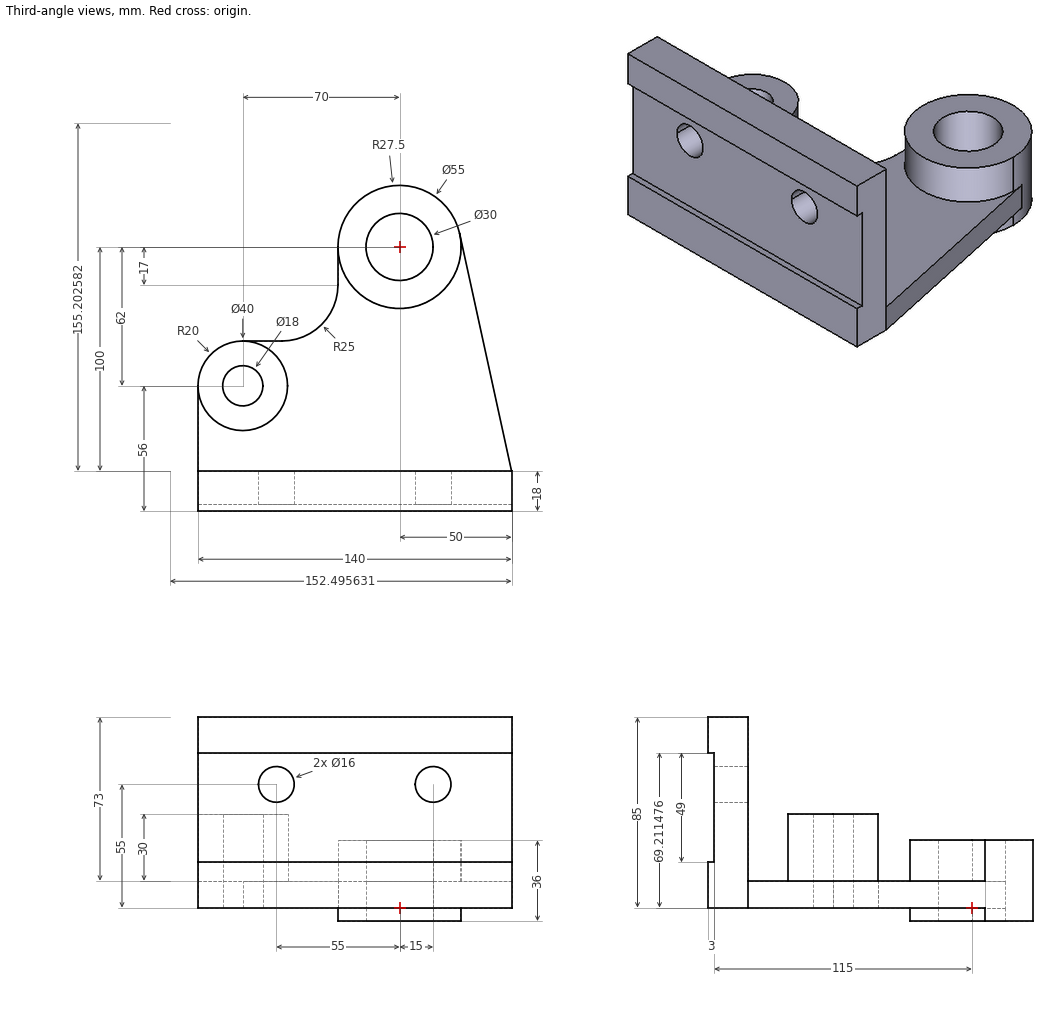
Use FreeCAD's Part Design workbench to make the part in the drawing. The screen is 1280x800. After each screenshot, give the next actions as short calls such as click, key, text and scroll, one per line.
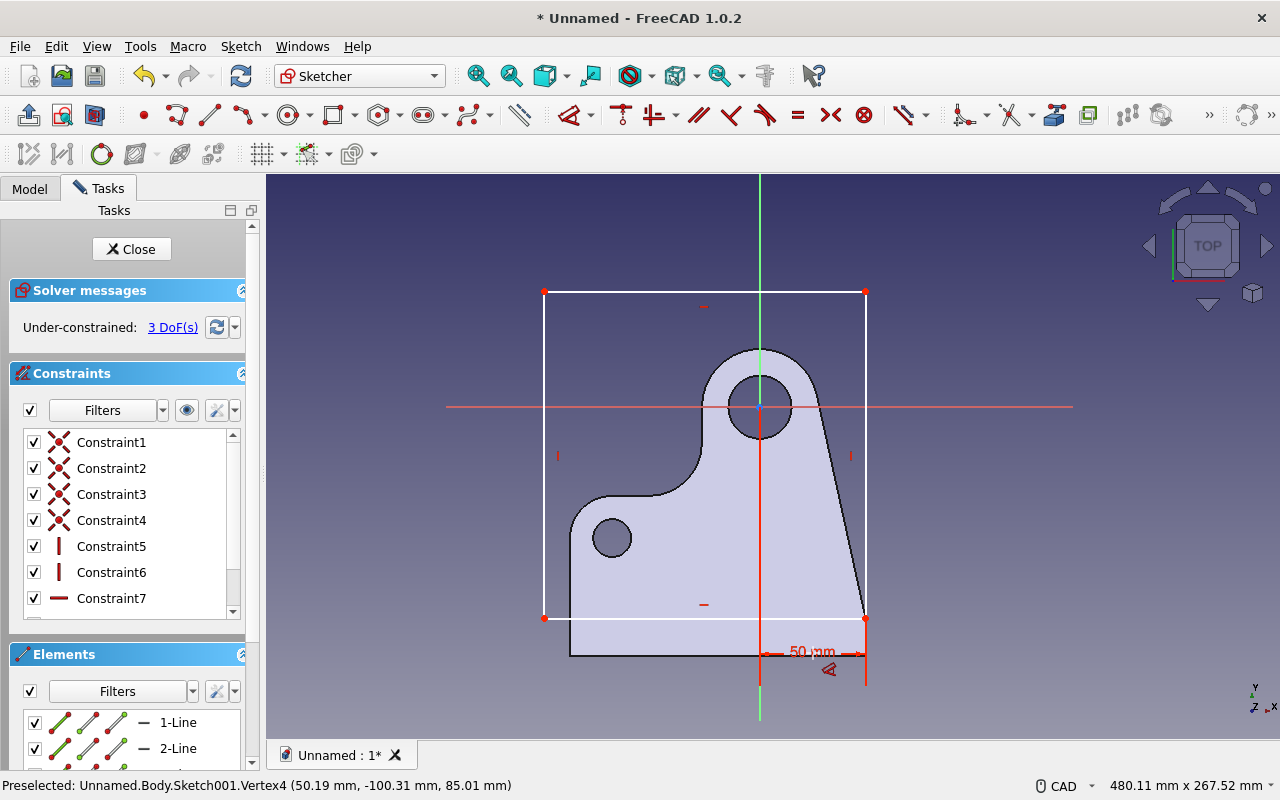
click(544, 619)
click(510, 513)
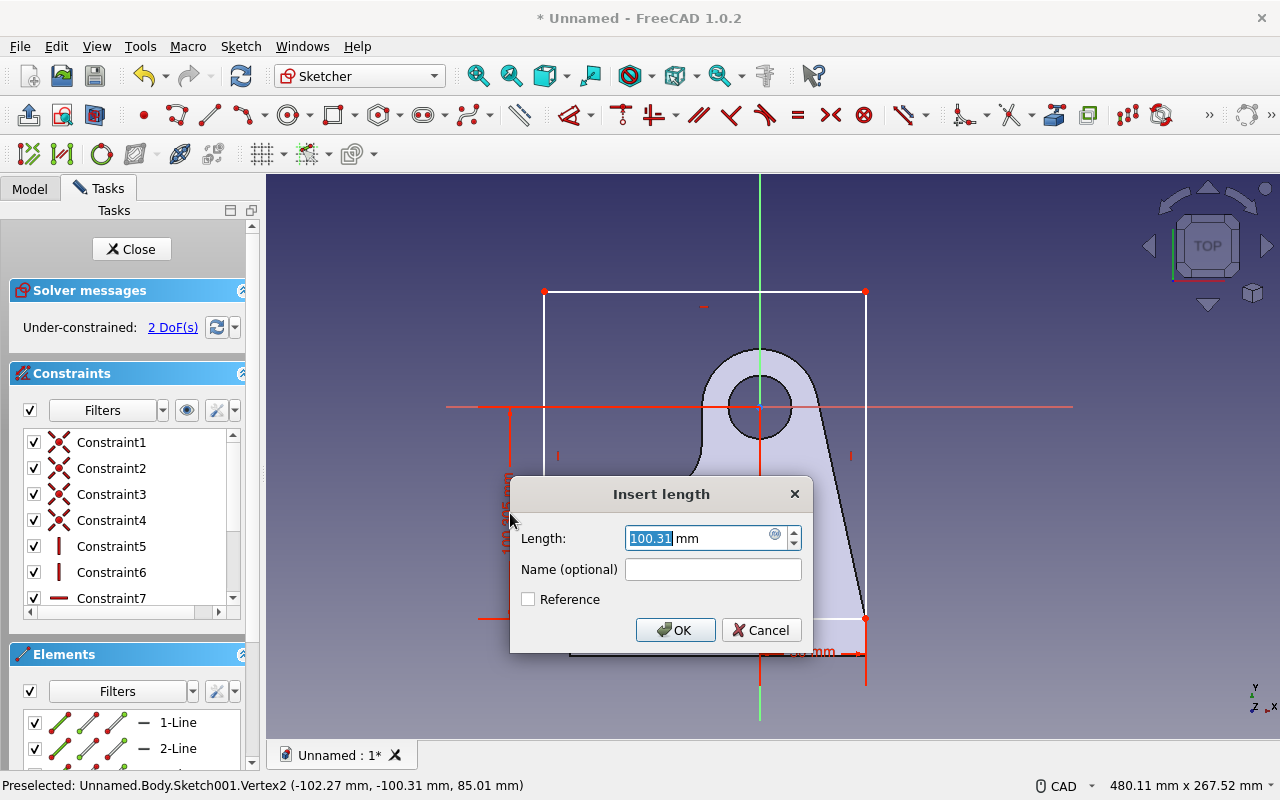
text(100)
key(Return)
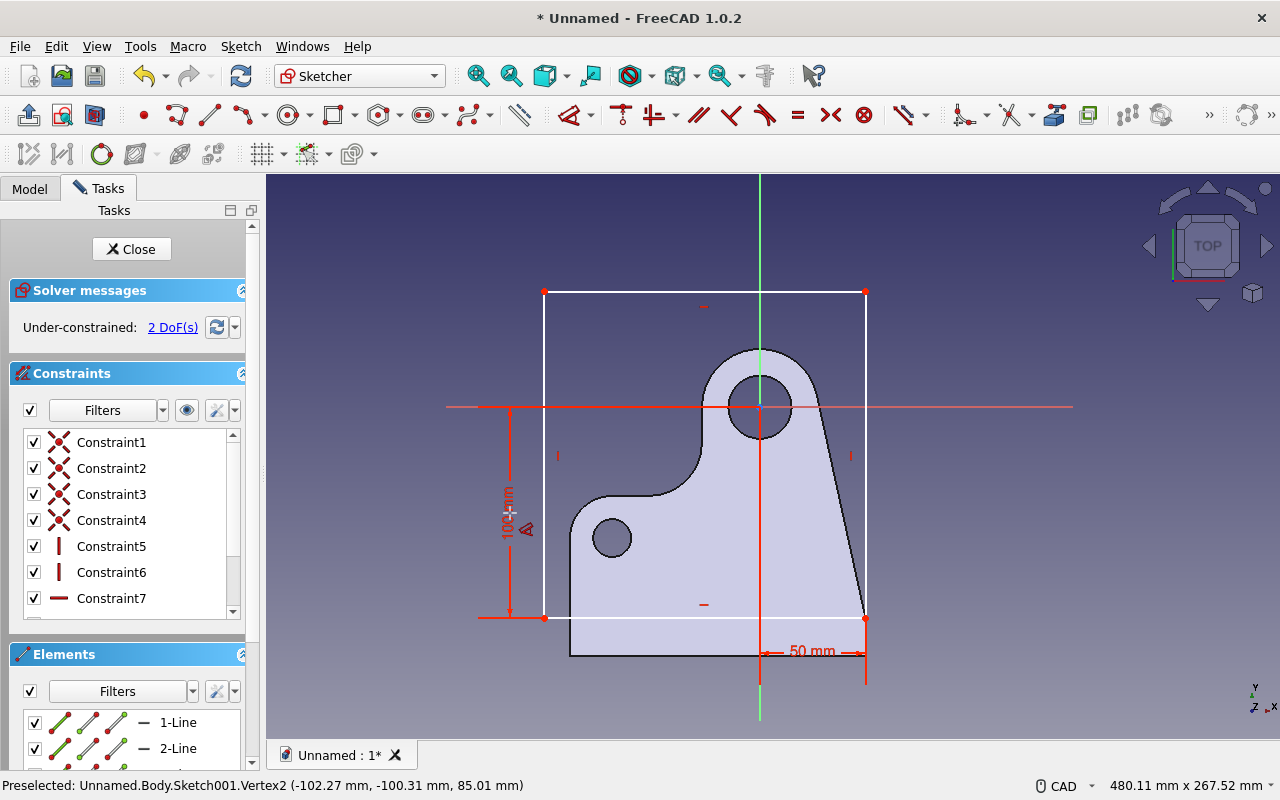
click(544, 390)
click(510, 455)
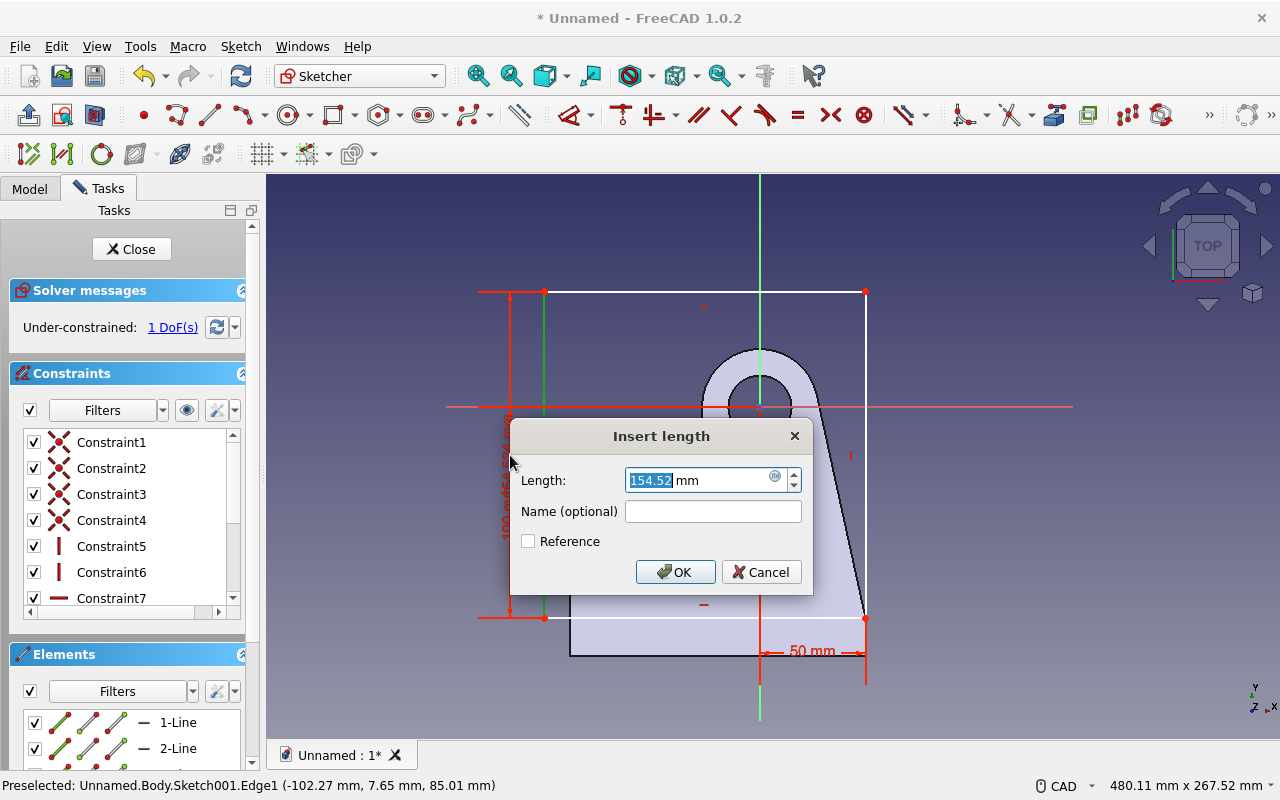
text(155.202582)
key(Return)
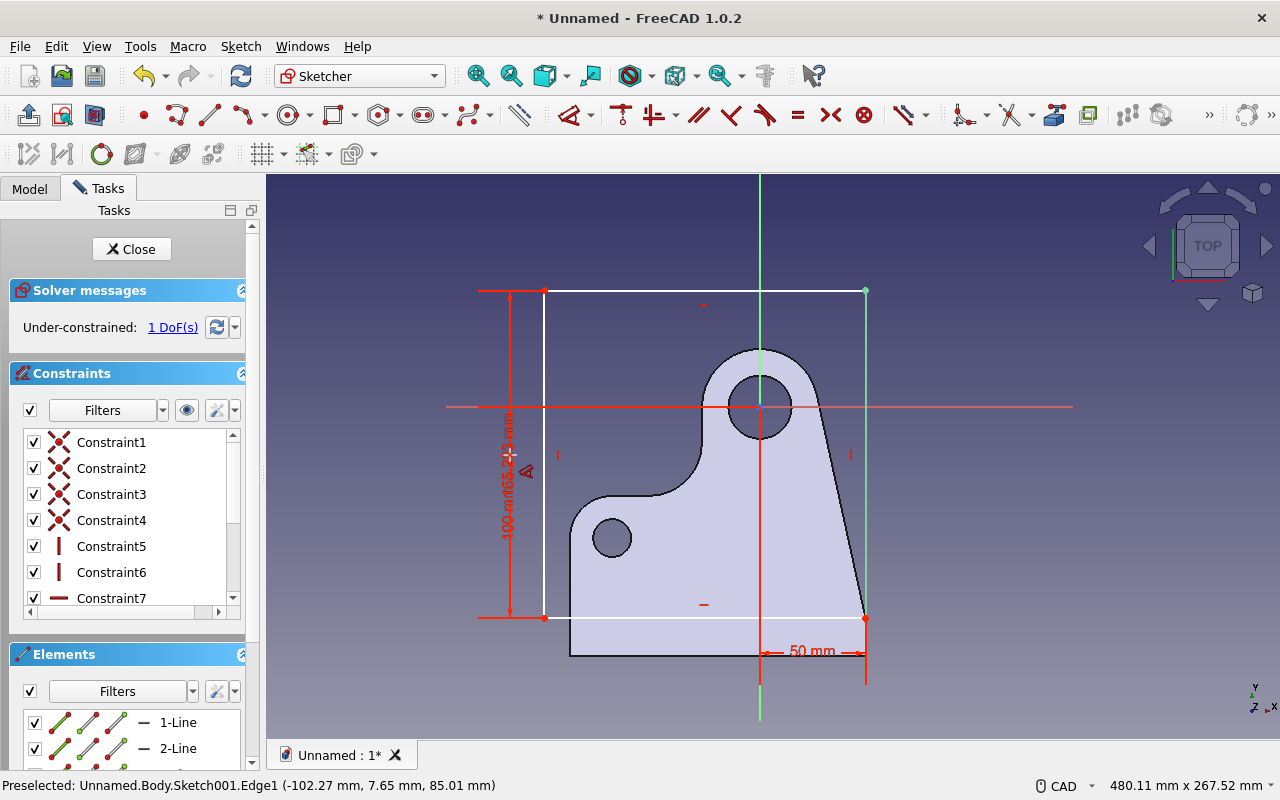
click(640, 618)
click(705, 652)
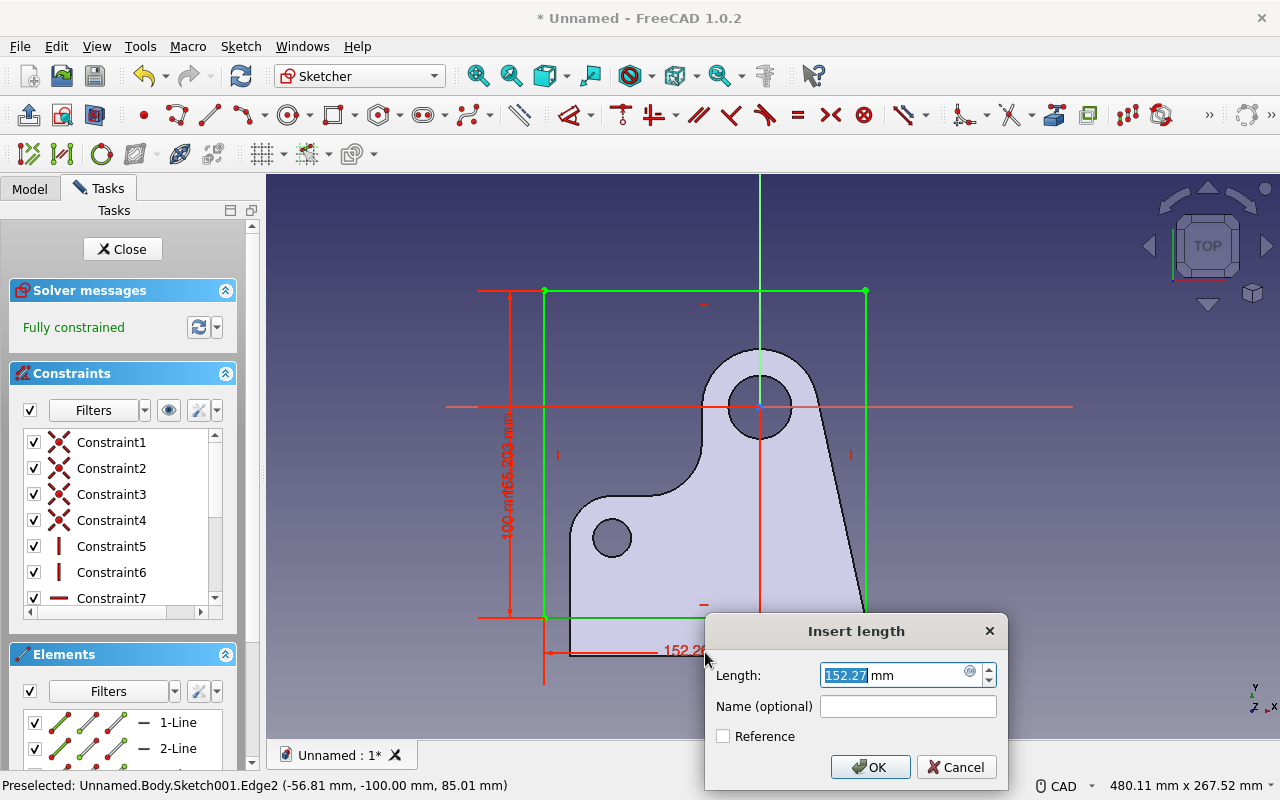
text(152.495631)
key(Return)
key(Escape)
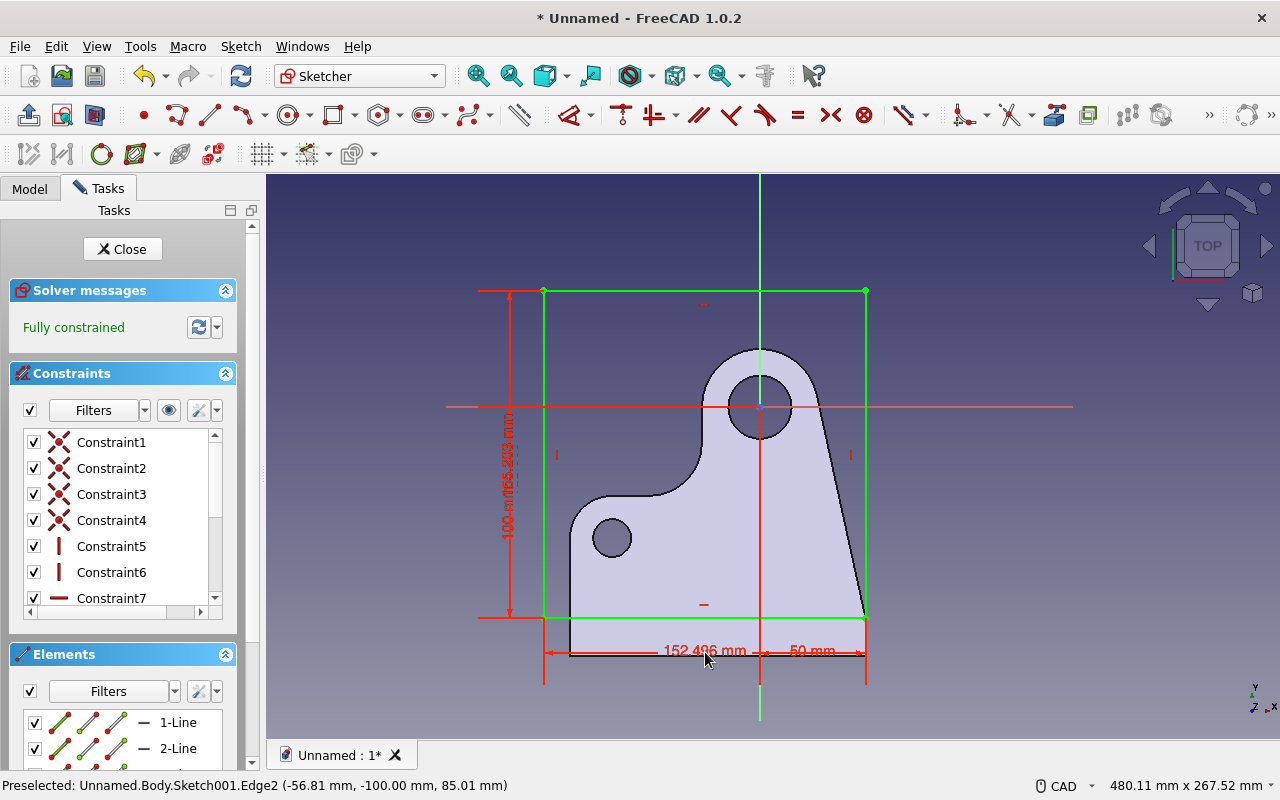
click(123, 249)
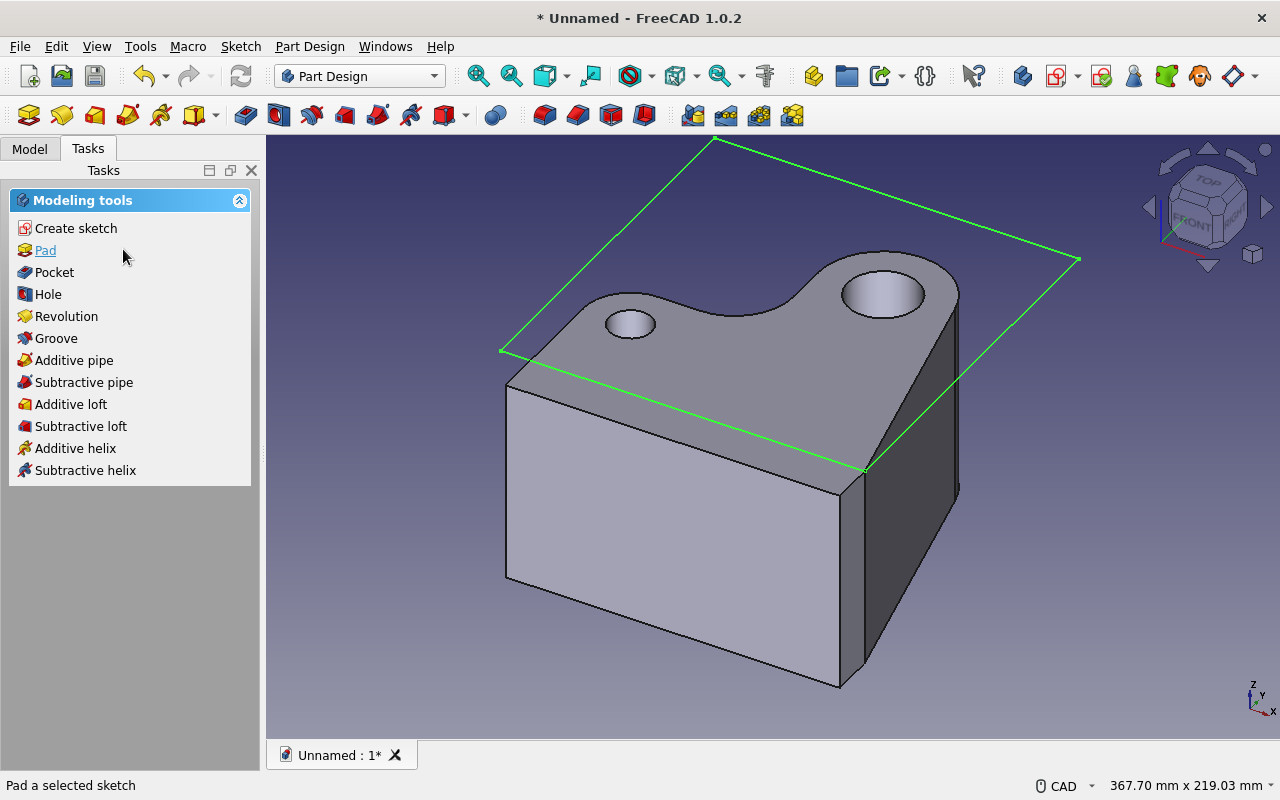
click(246, 116)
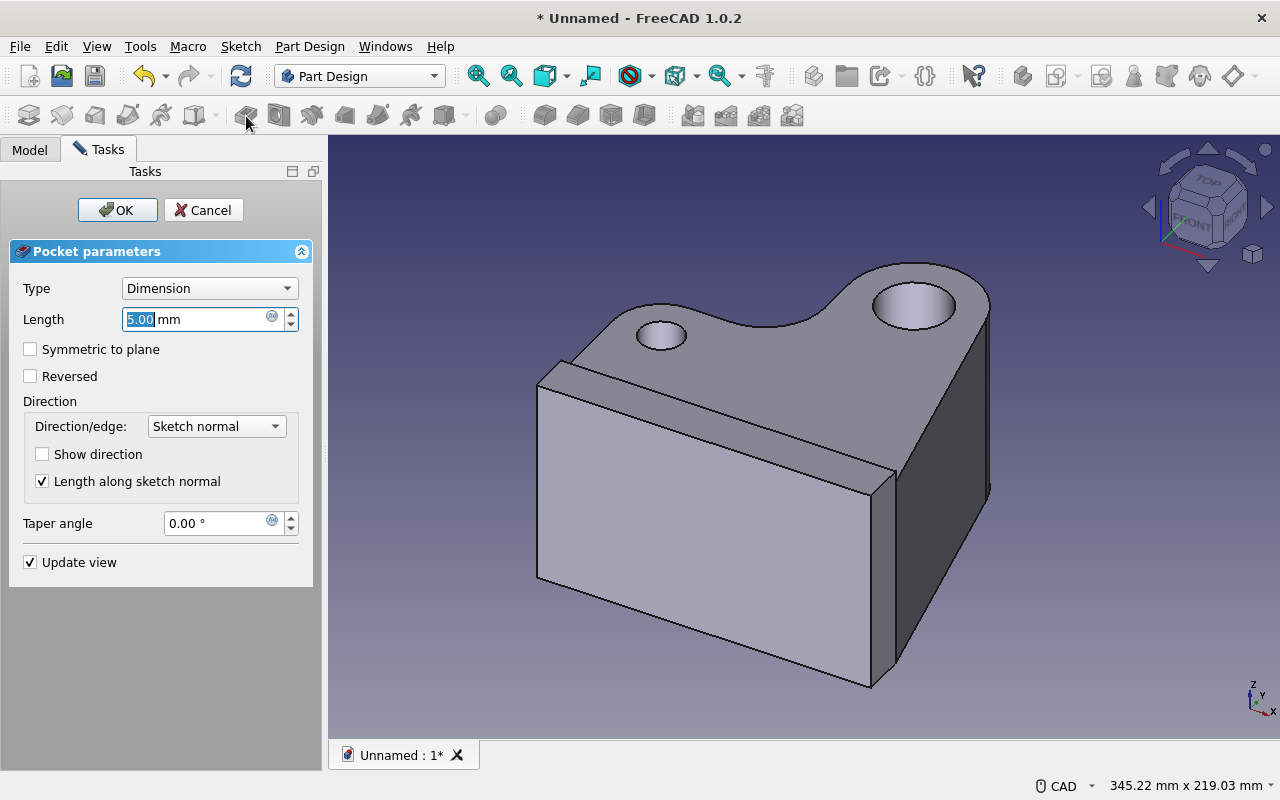
text(73)
key(Tab)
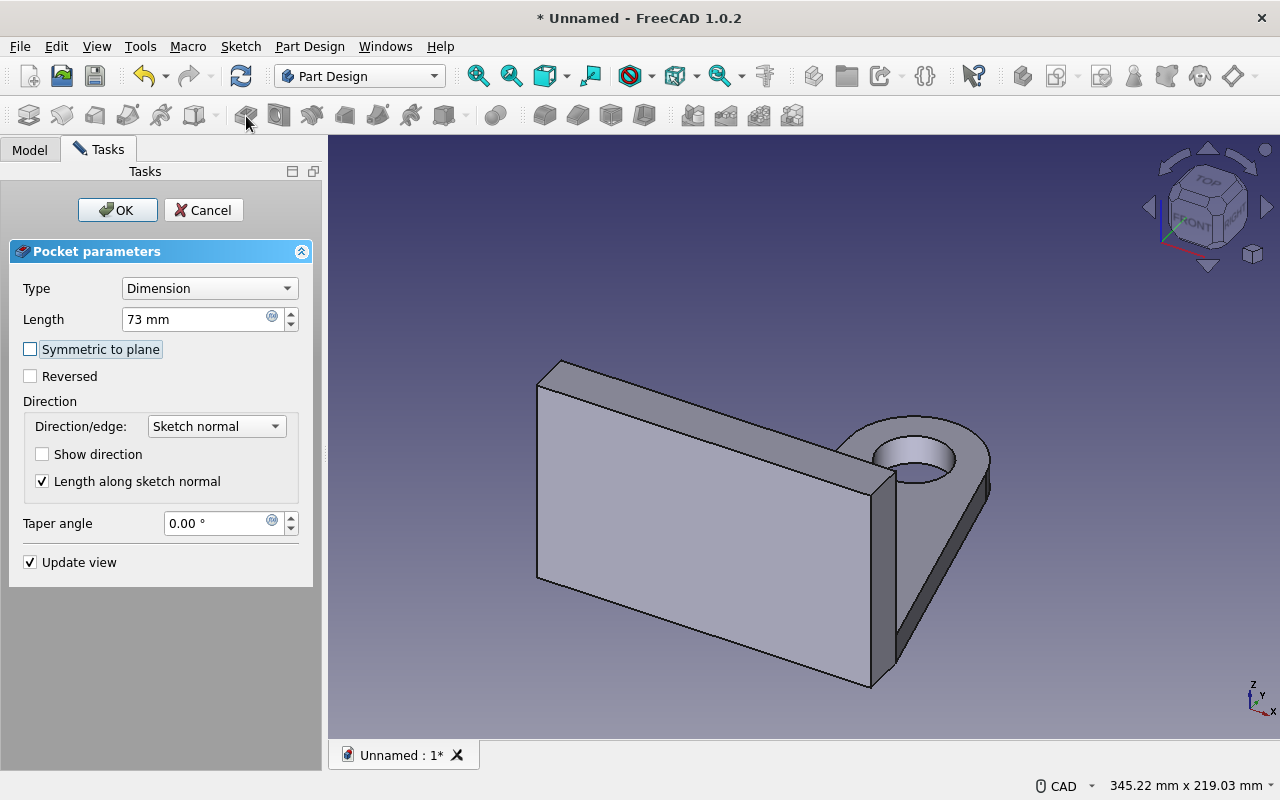
click(118, 210)